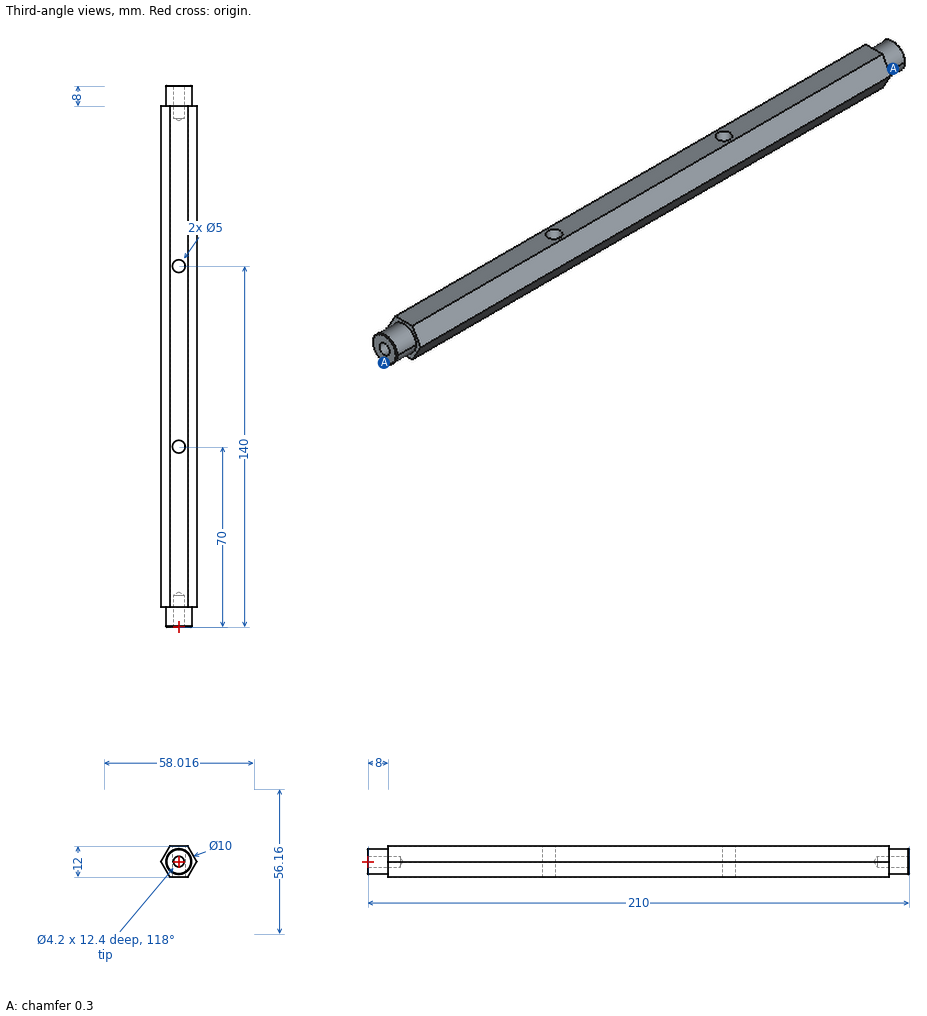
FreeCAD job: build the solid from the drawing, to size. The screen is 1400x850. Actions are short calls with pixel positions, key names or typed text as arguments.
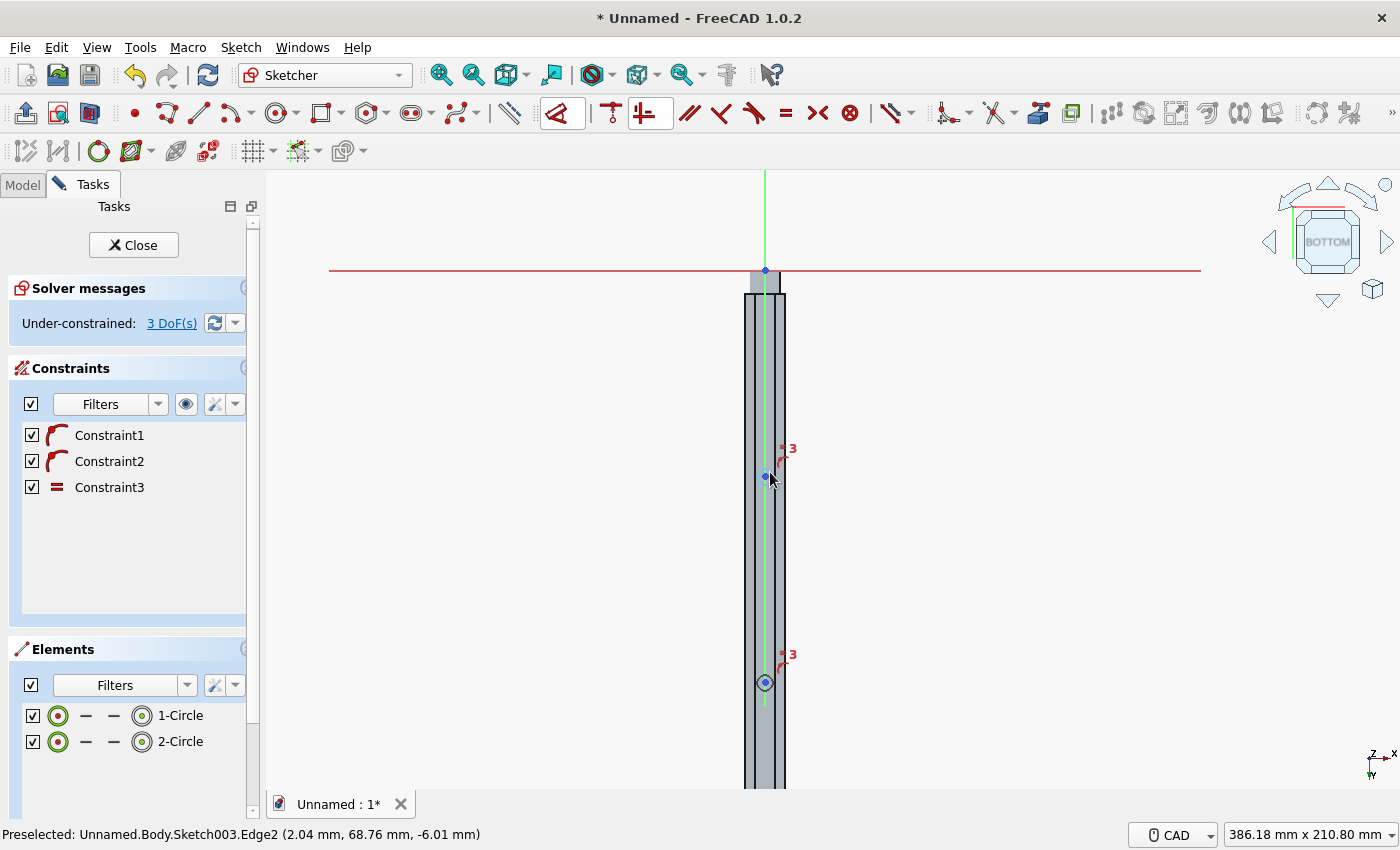
scroll(770, 678, up, 5)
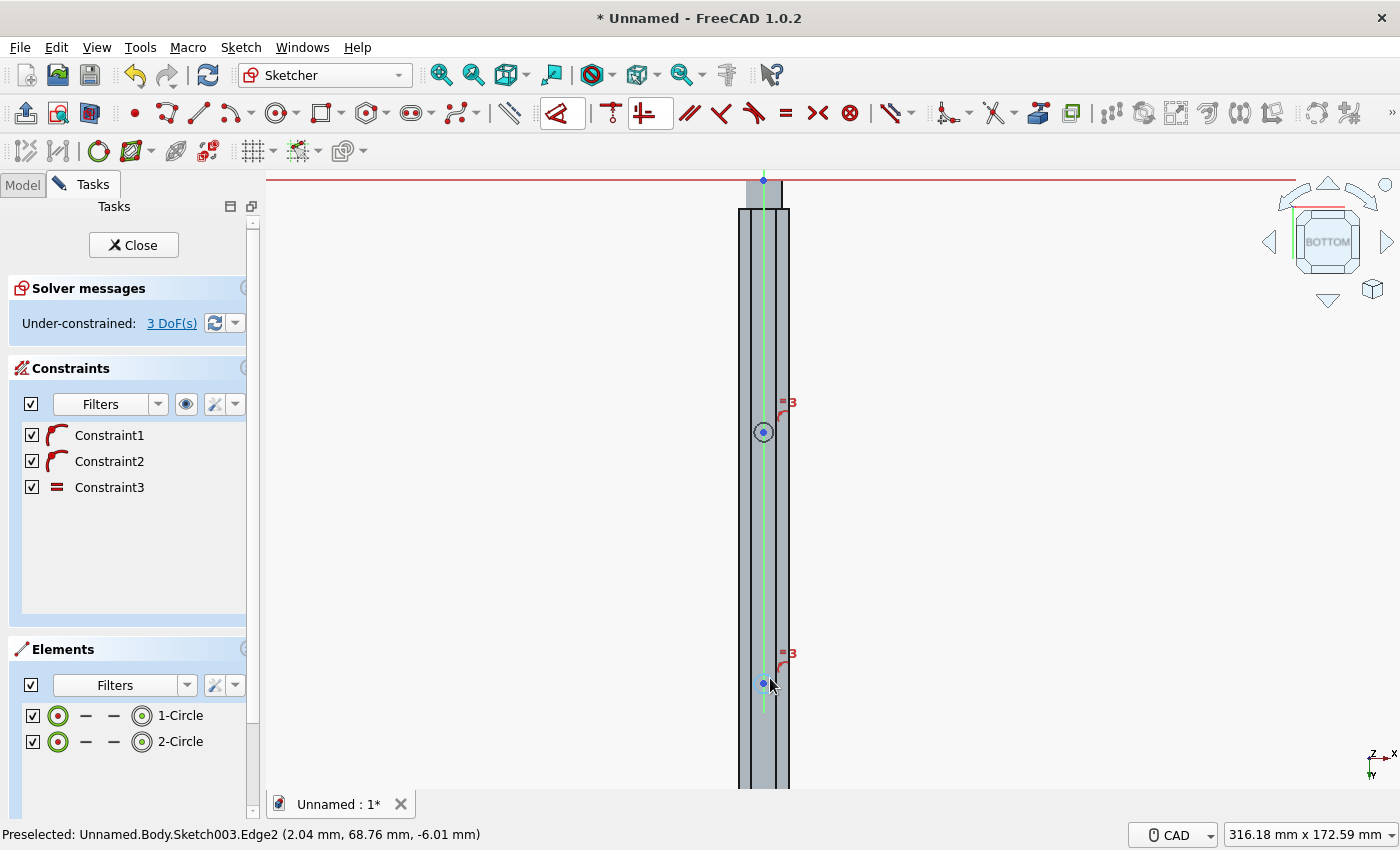
click(770, 675)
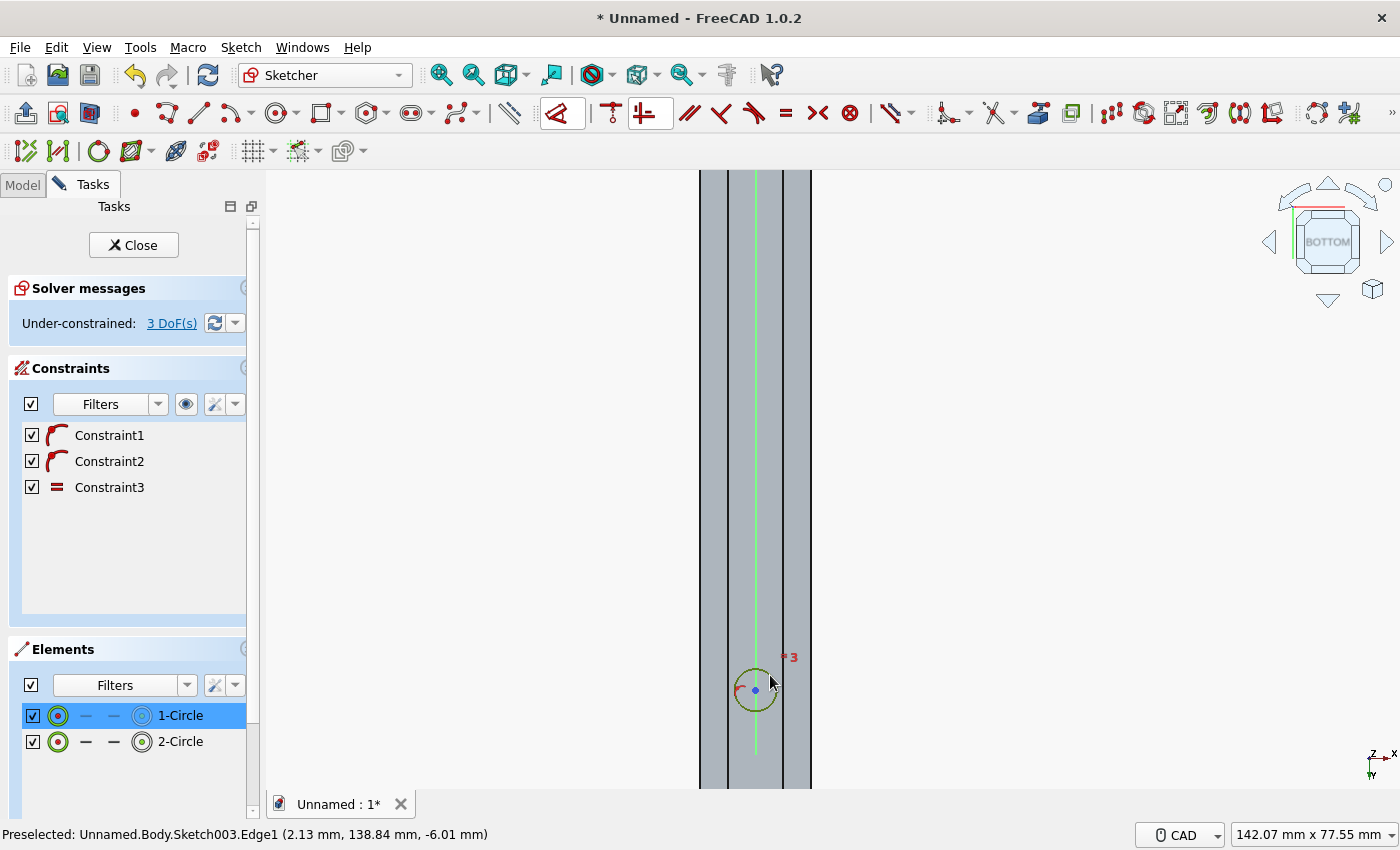
key(k)
key(o)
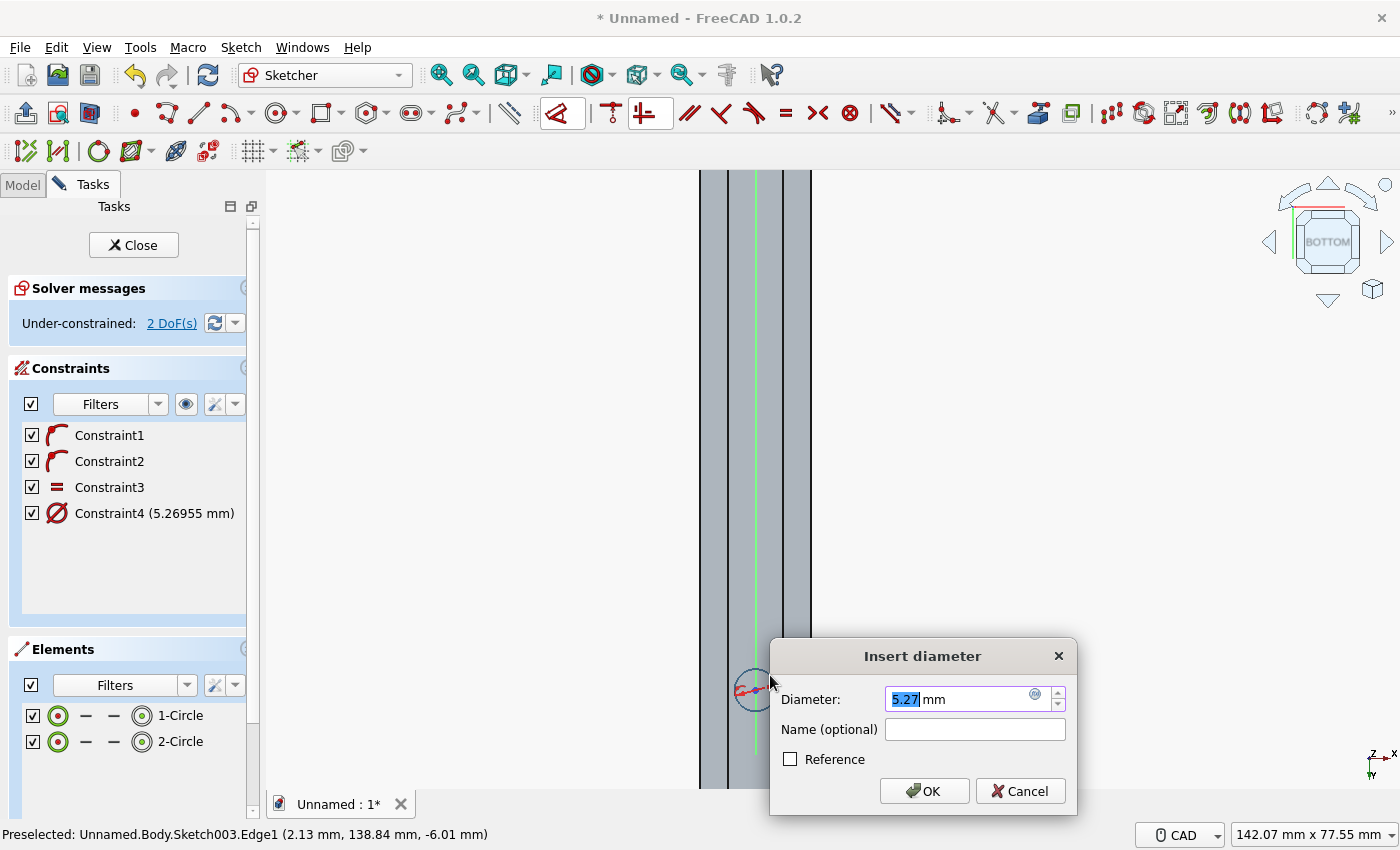
text(5)
key(Return)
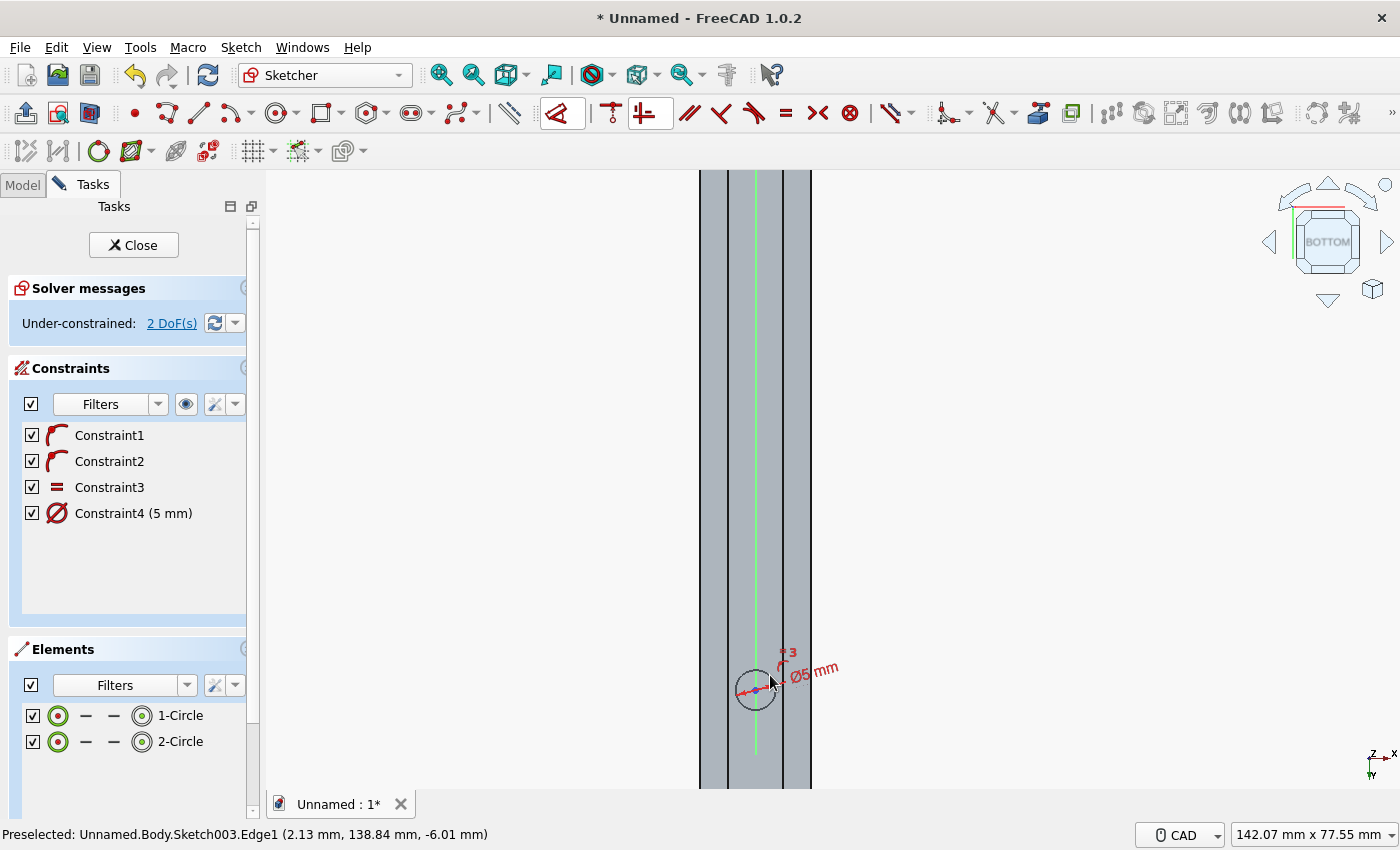
scroll(770, 678, down, 5)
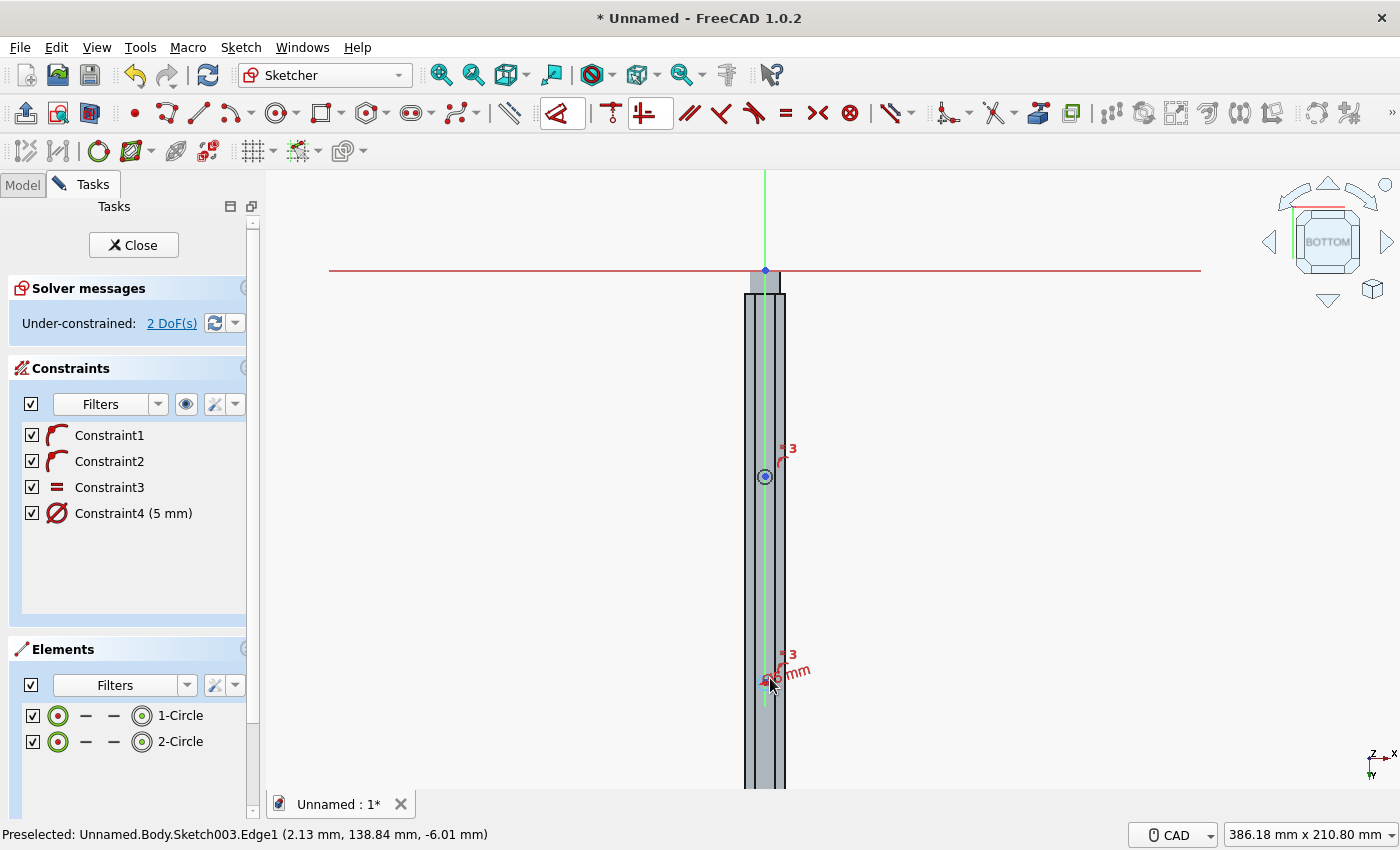
click(765, 477)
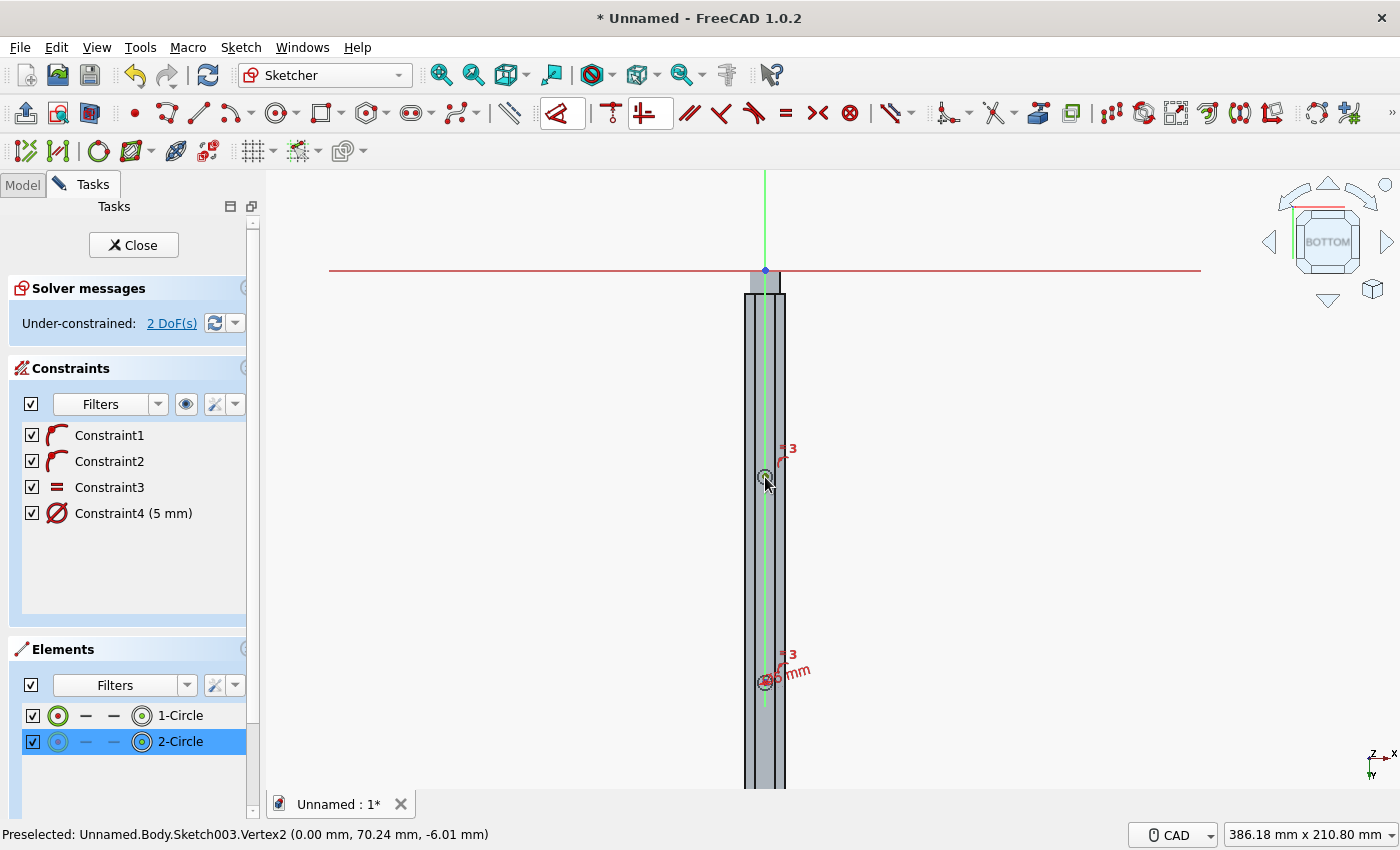
key(i)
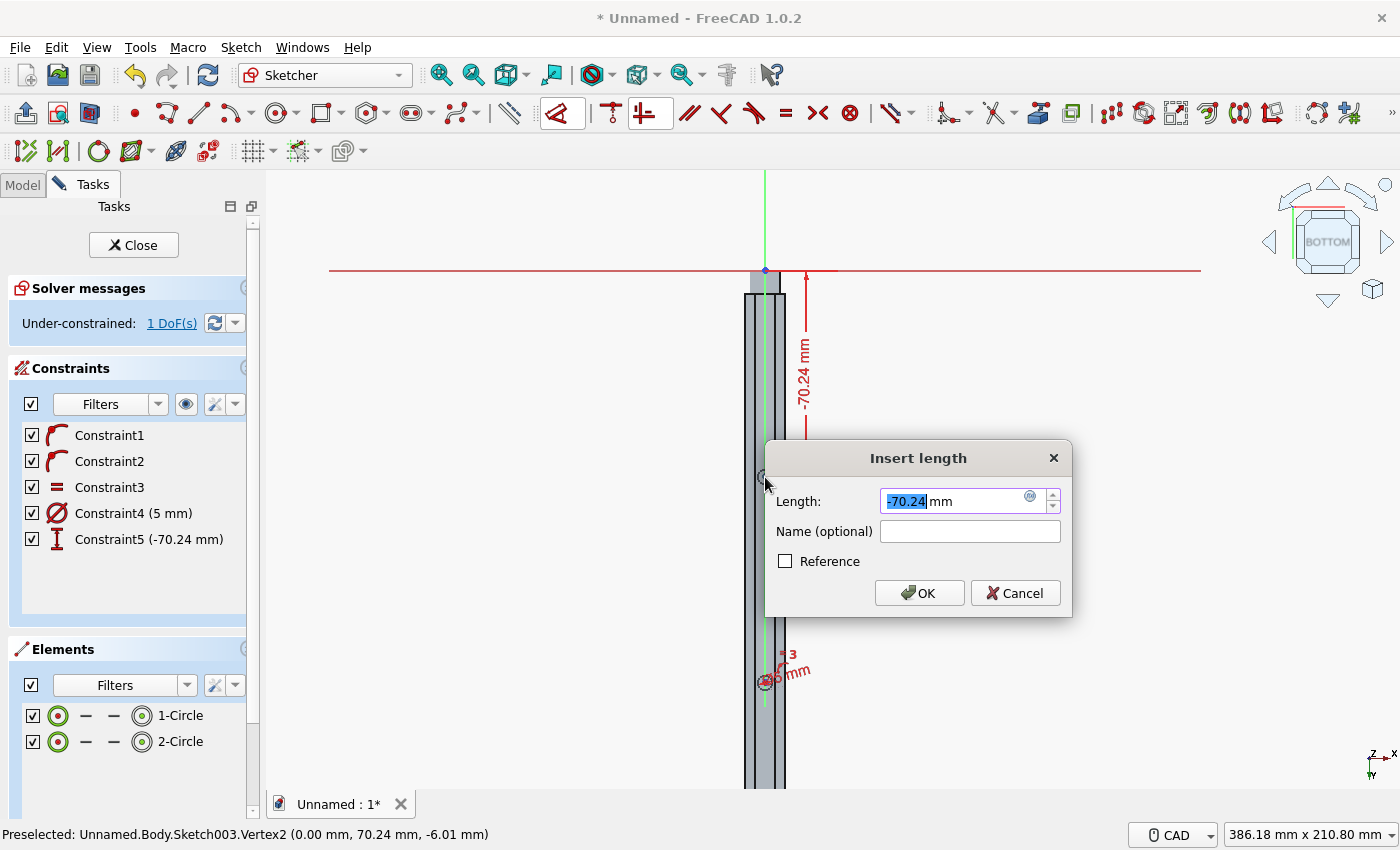
text(-70)
key(Return)